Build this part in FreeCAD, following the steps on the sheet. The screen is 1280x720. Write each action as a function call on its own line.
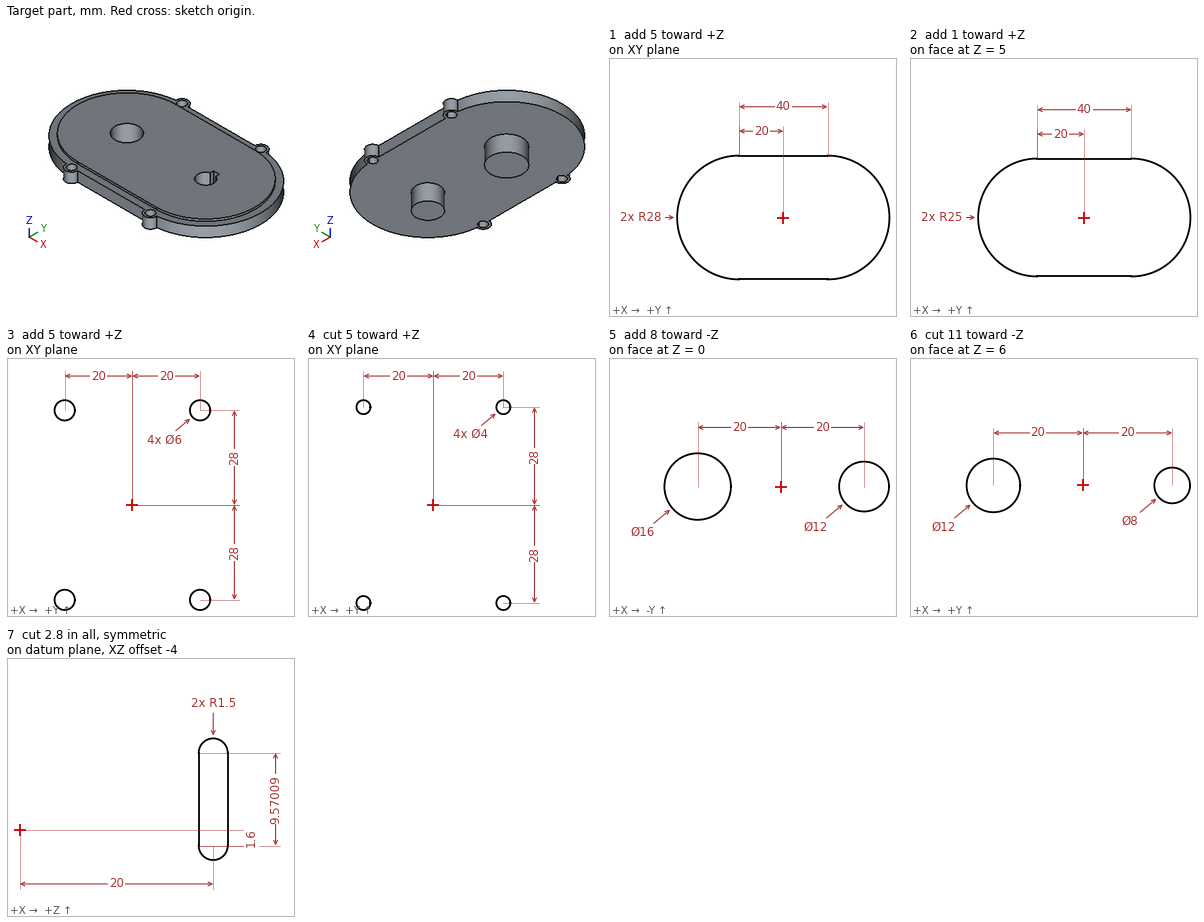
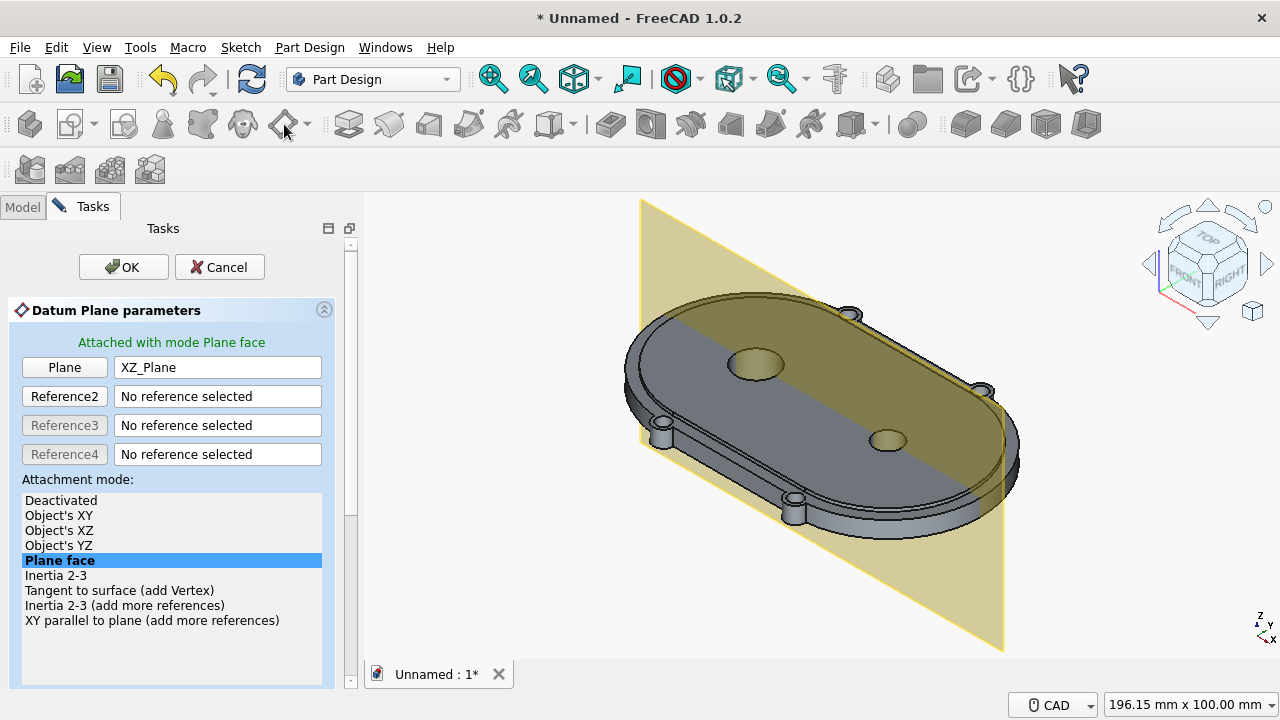
scroll(351, 463, down, 3)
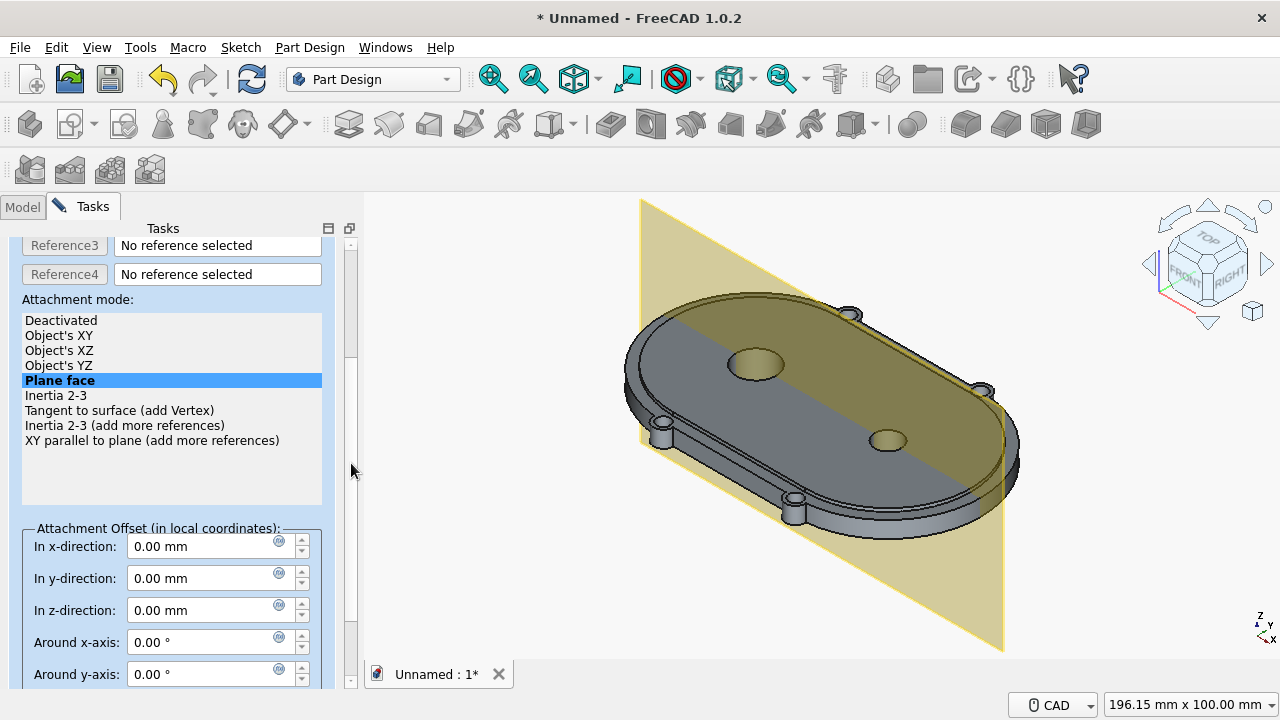
triple_click(210, 610)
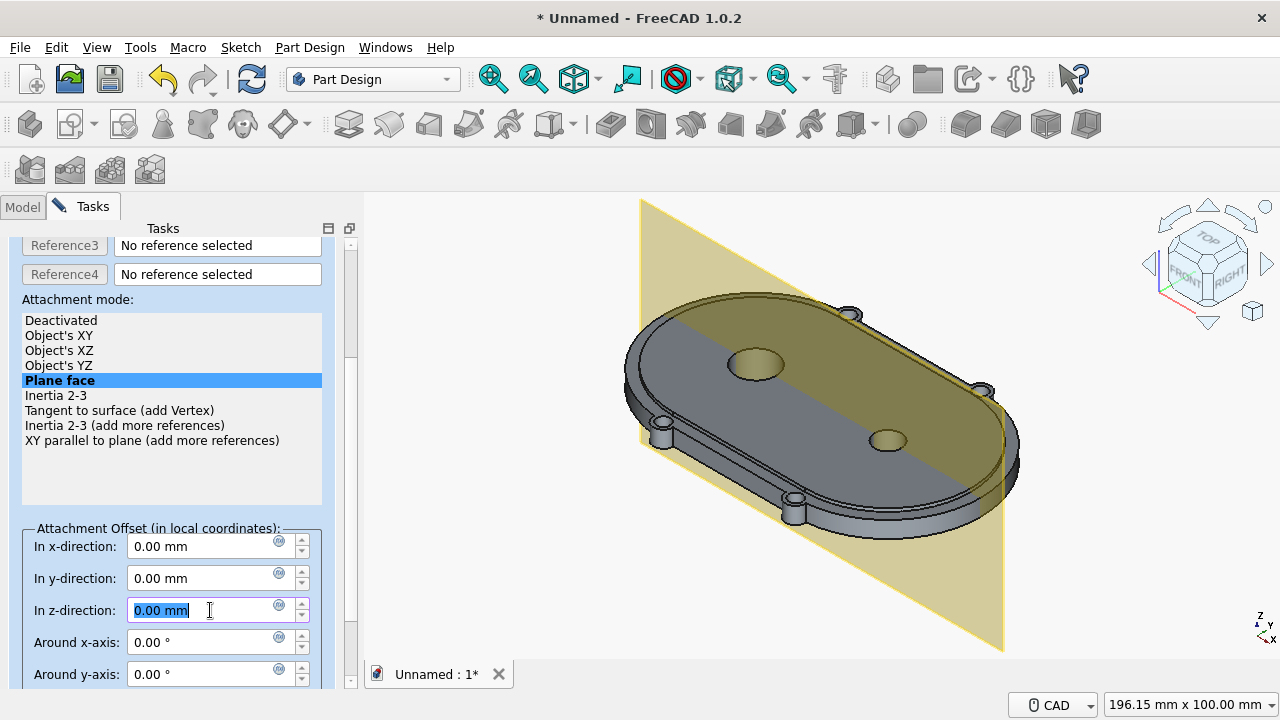
text(-4)
key(Tab)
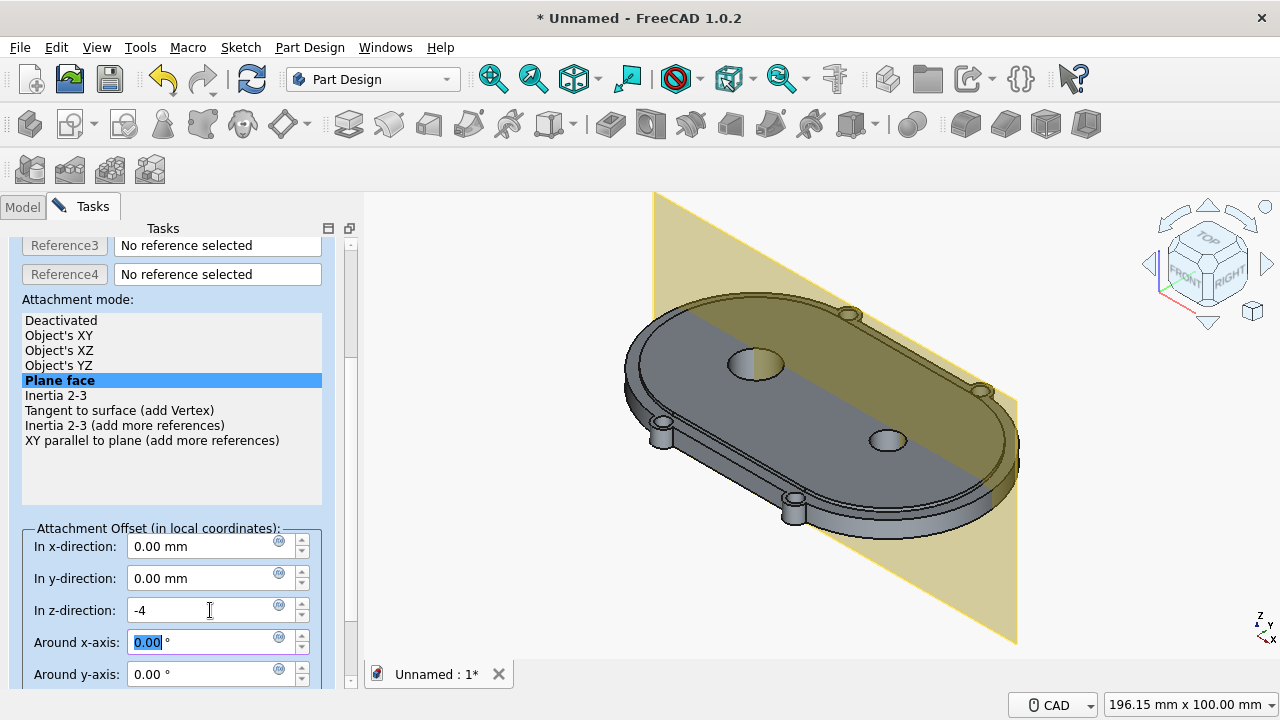
scroll(351, 463, up, 4)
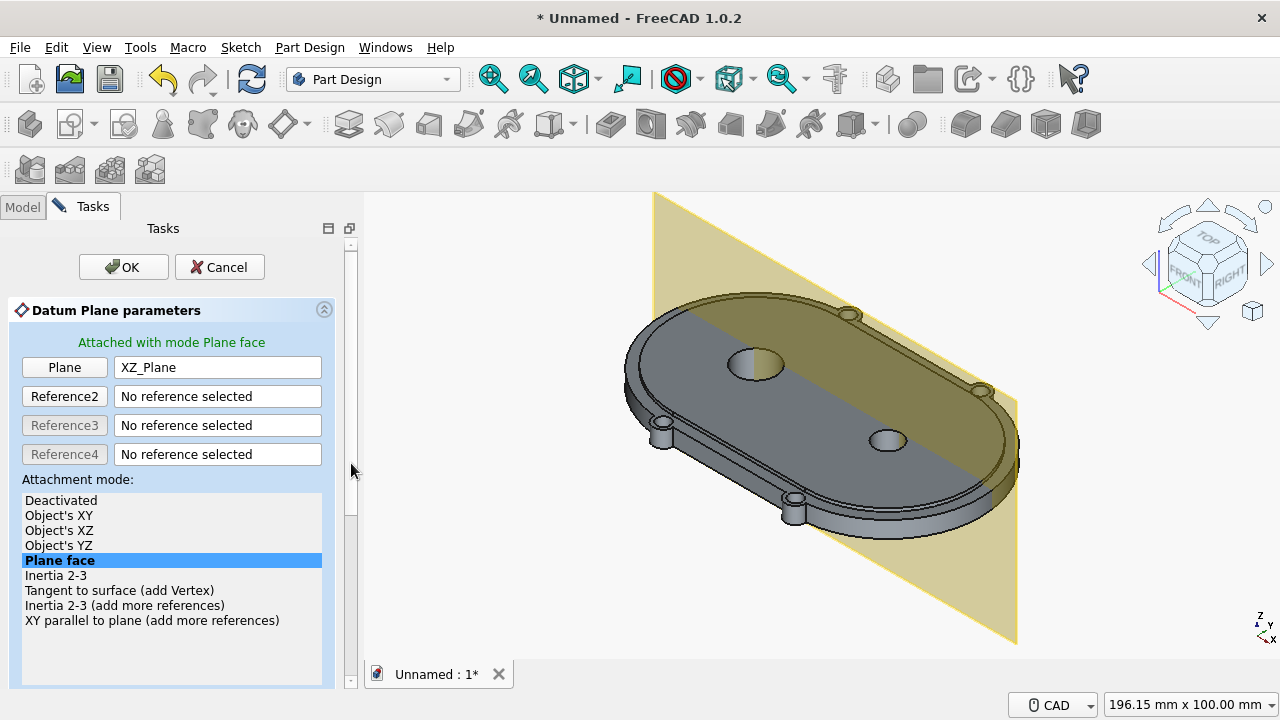
click(124, 267)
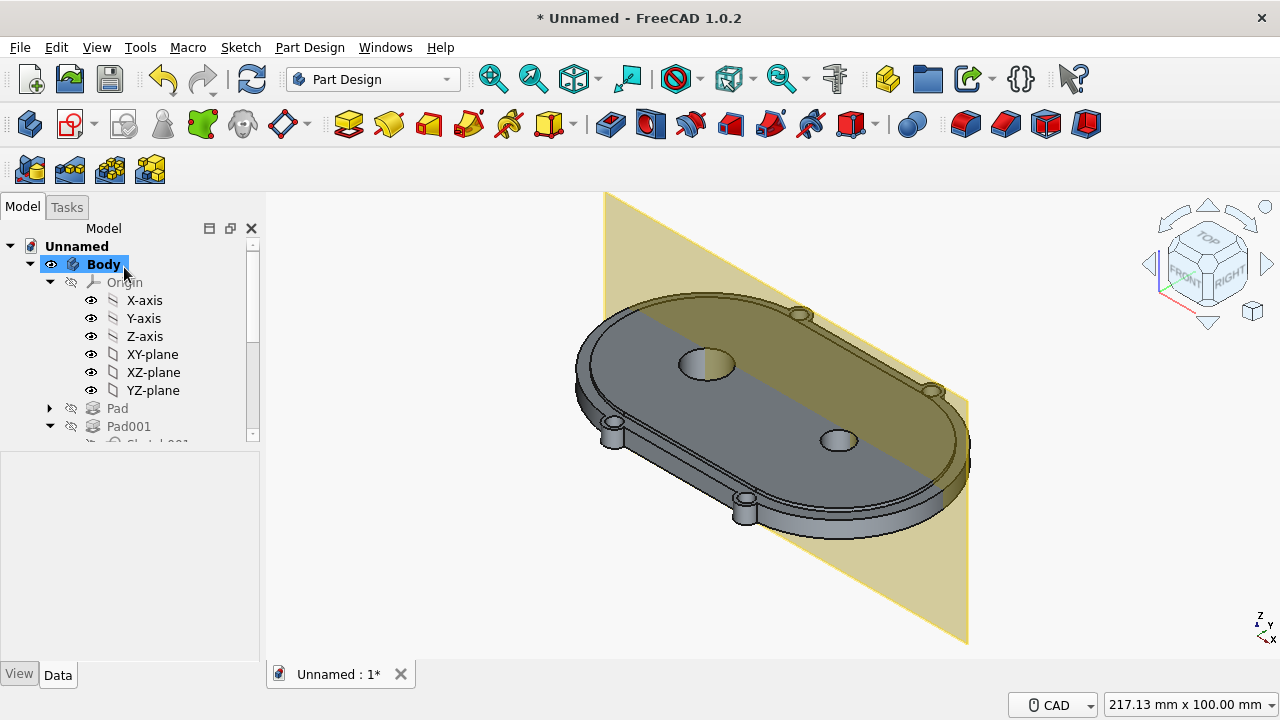
scroll(100, 332, down, 3)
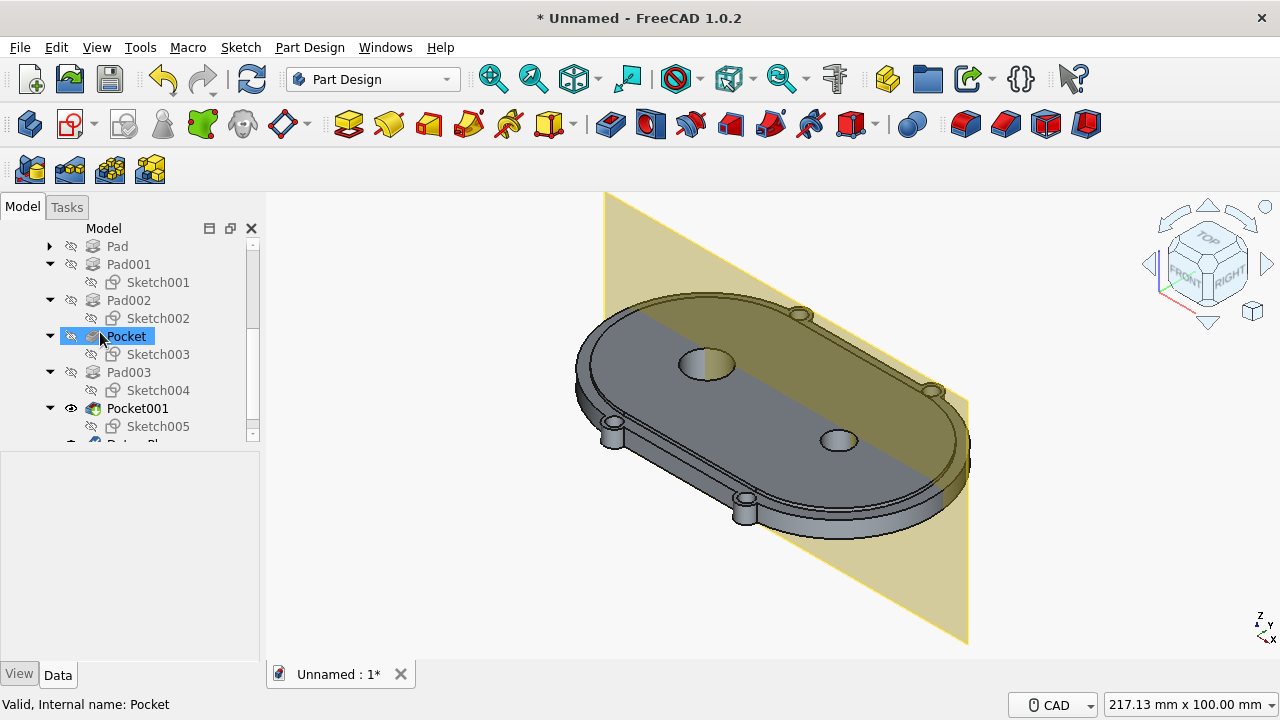
scroll(140, 332, up, 15)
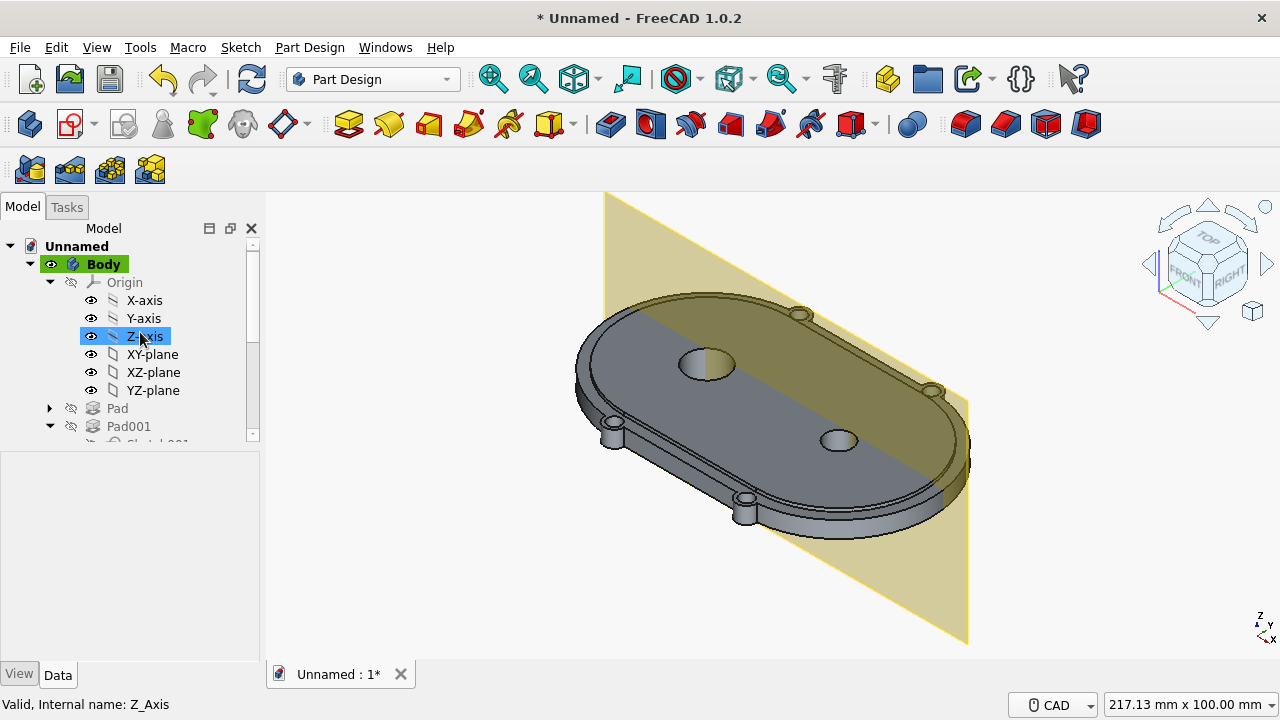
scroll(100, 332, down, 6)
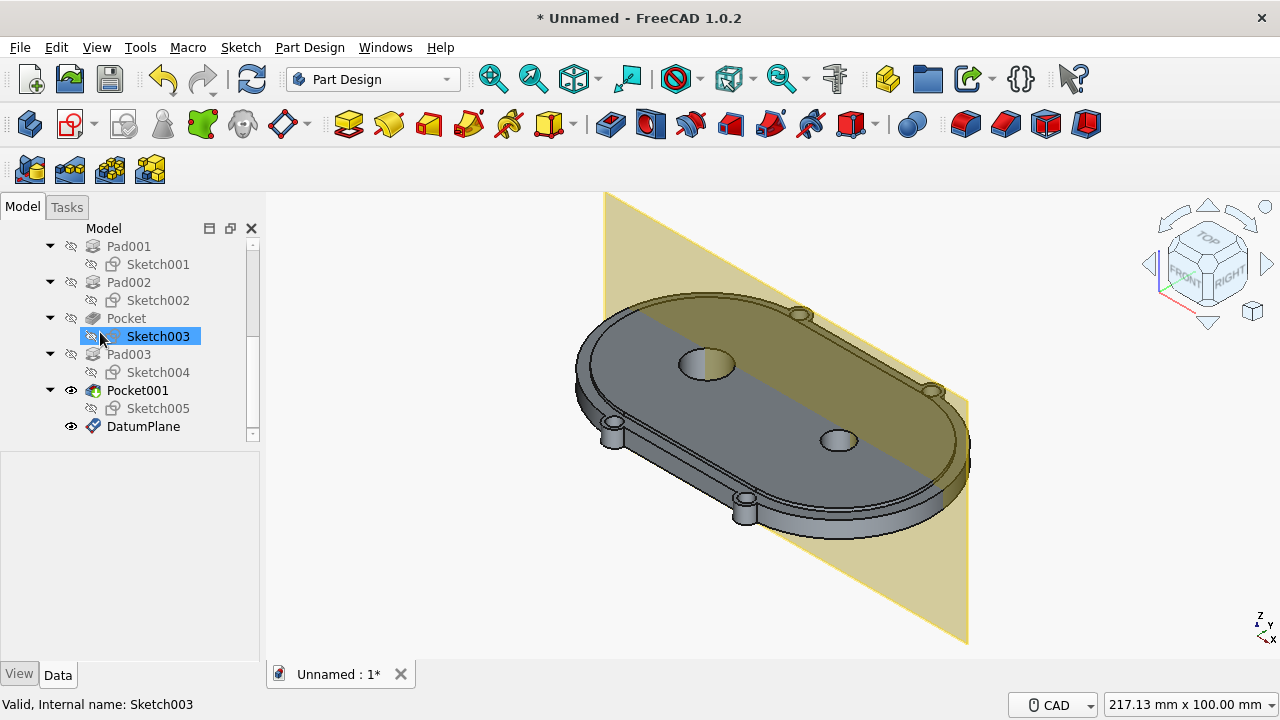
click(116, 426)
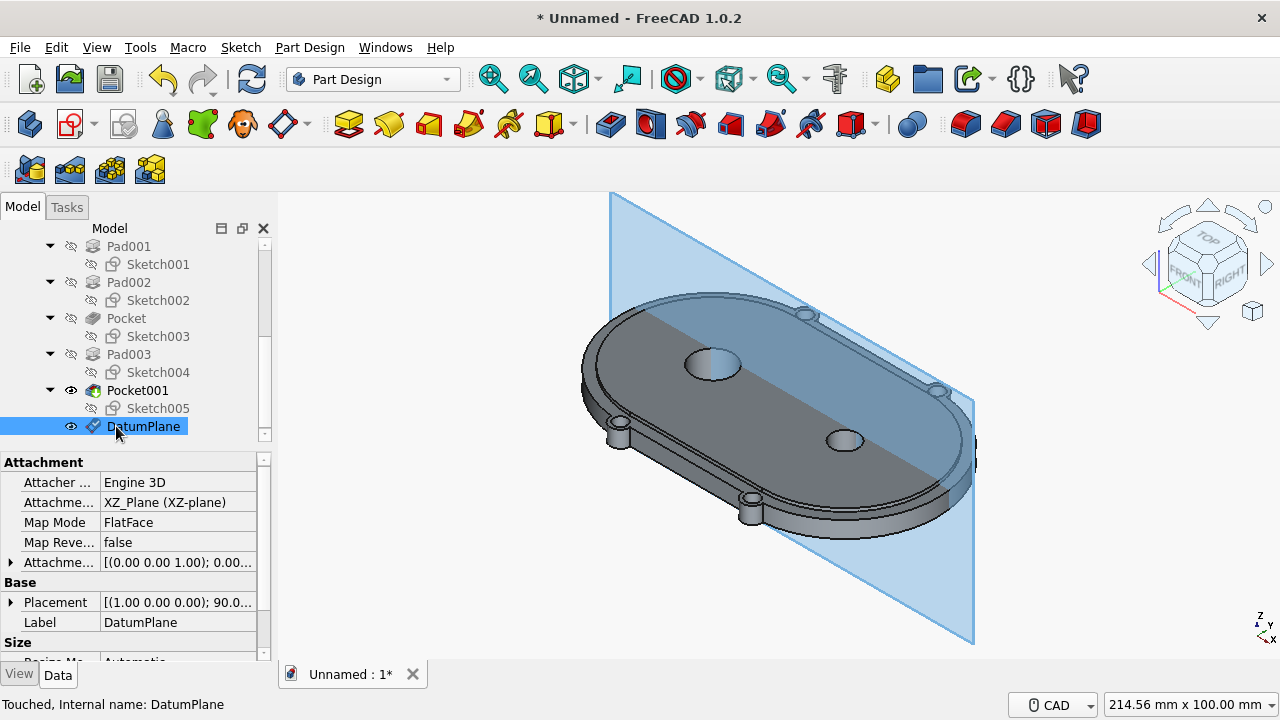
click(70, 124)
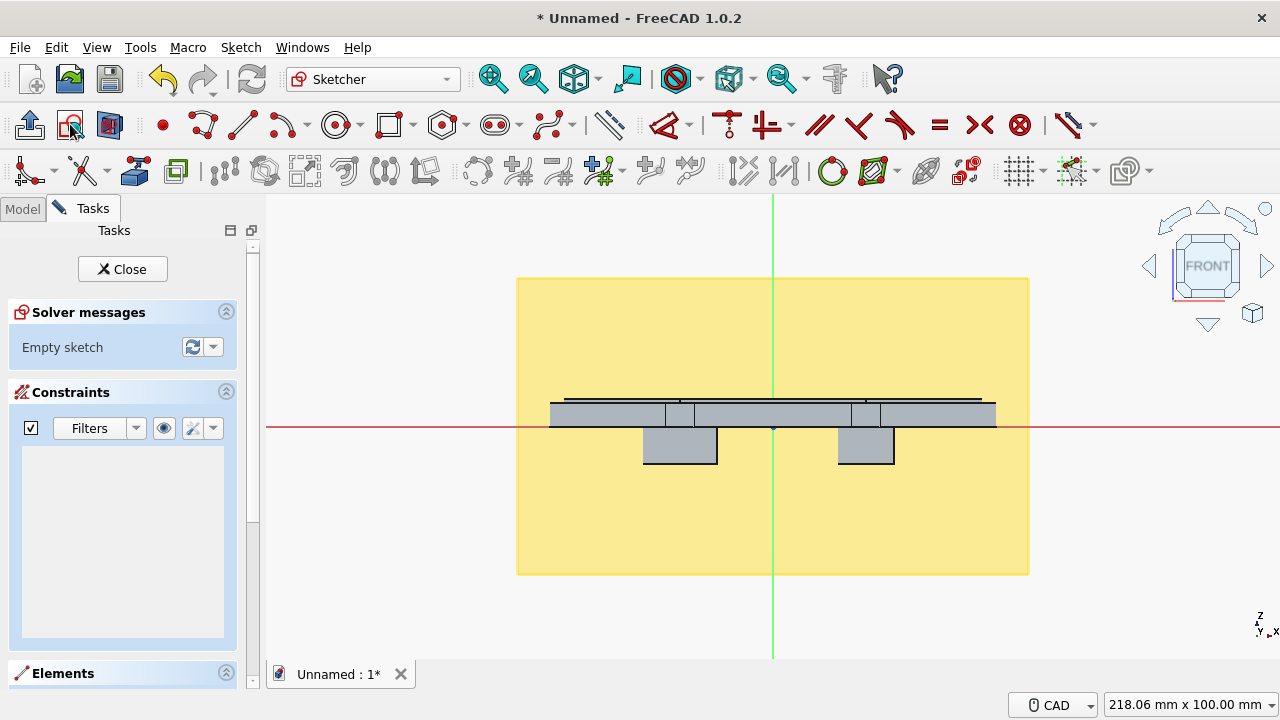
key(q)
key(s)